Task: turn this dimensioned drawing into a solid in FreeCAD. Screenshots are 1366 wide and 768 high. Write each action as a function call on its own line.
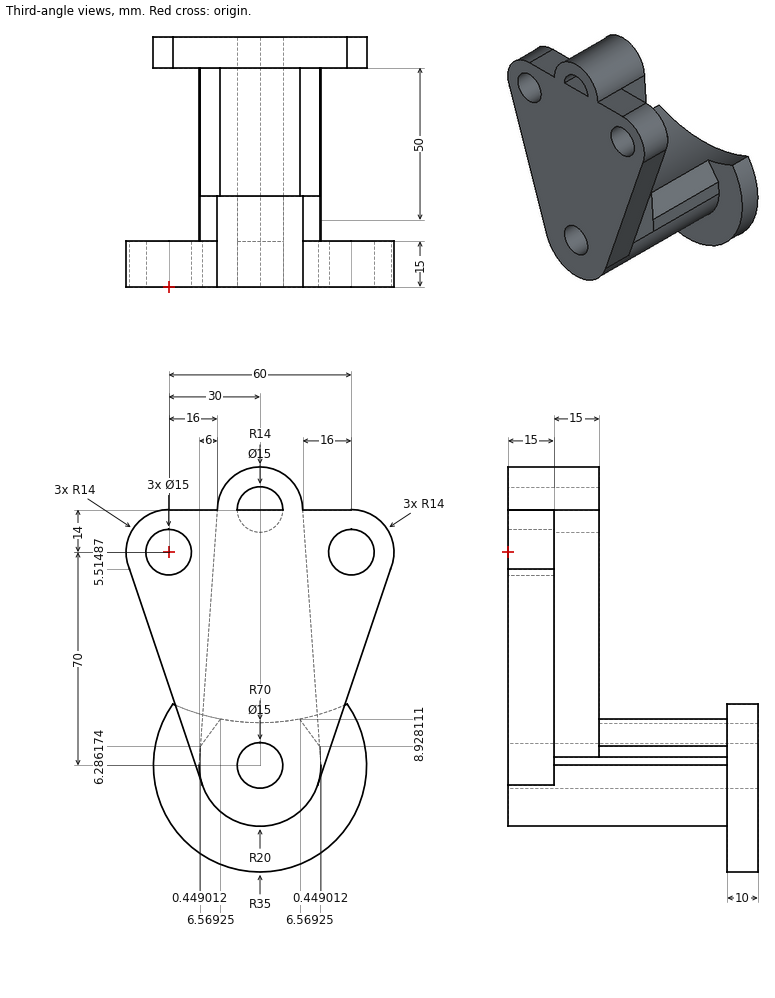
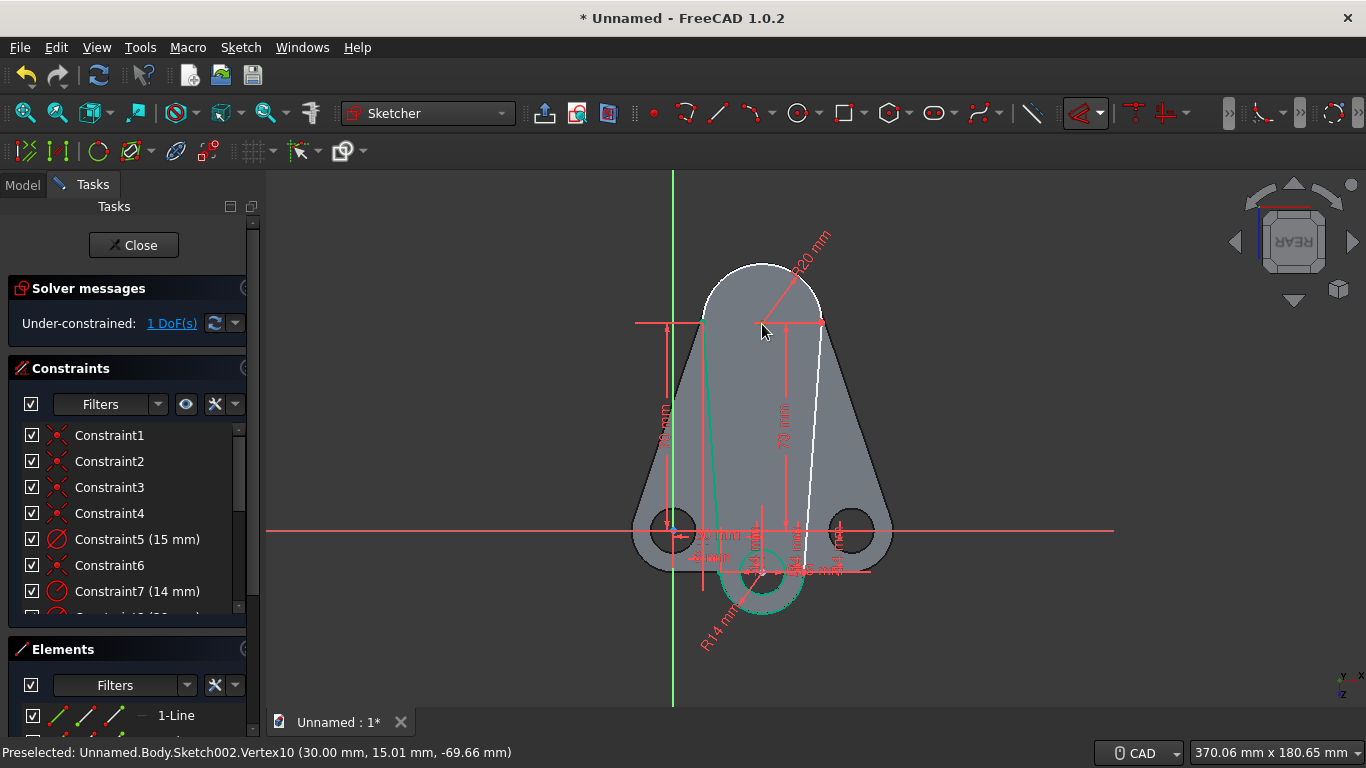
click(1102, 114)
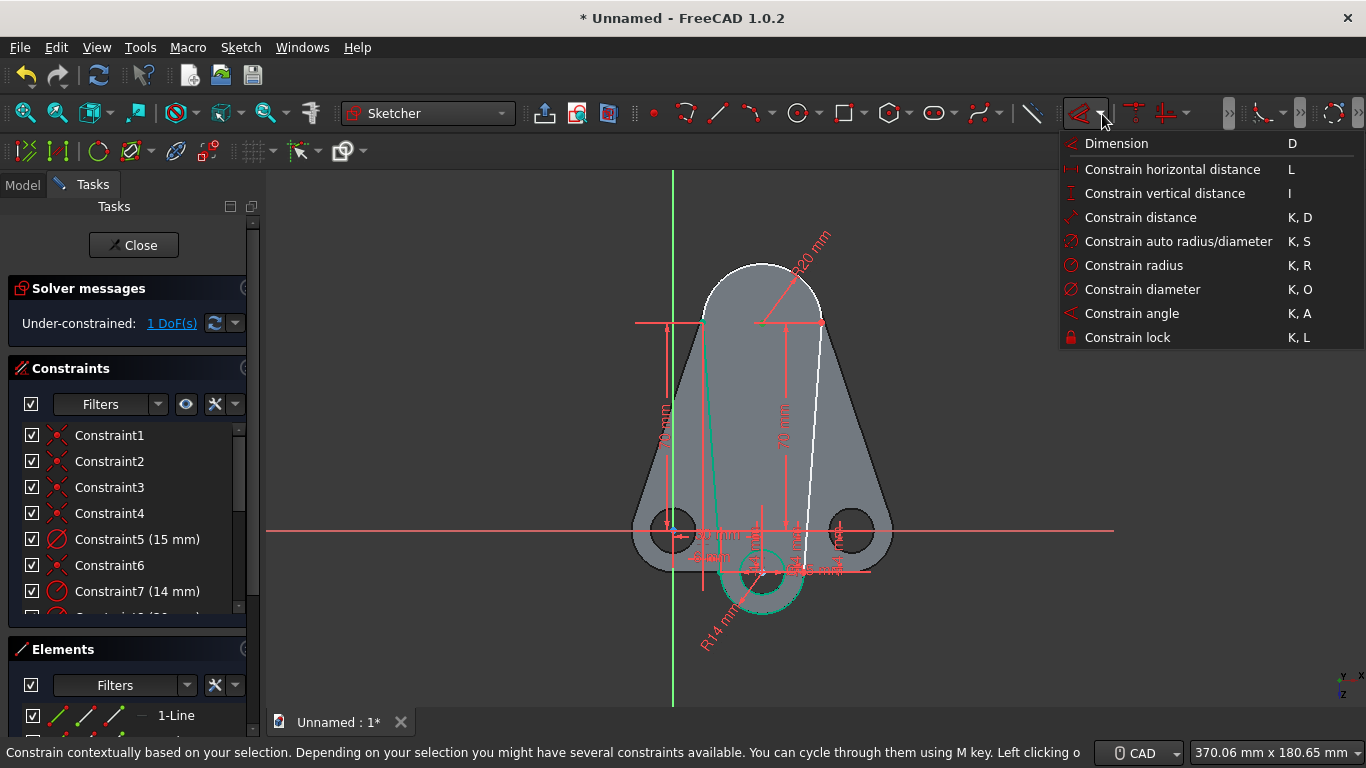
click(1212, 193)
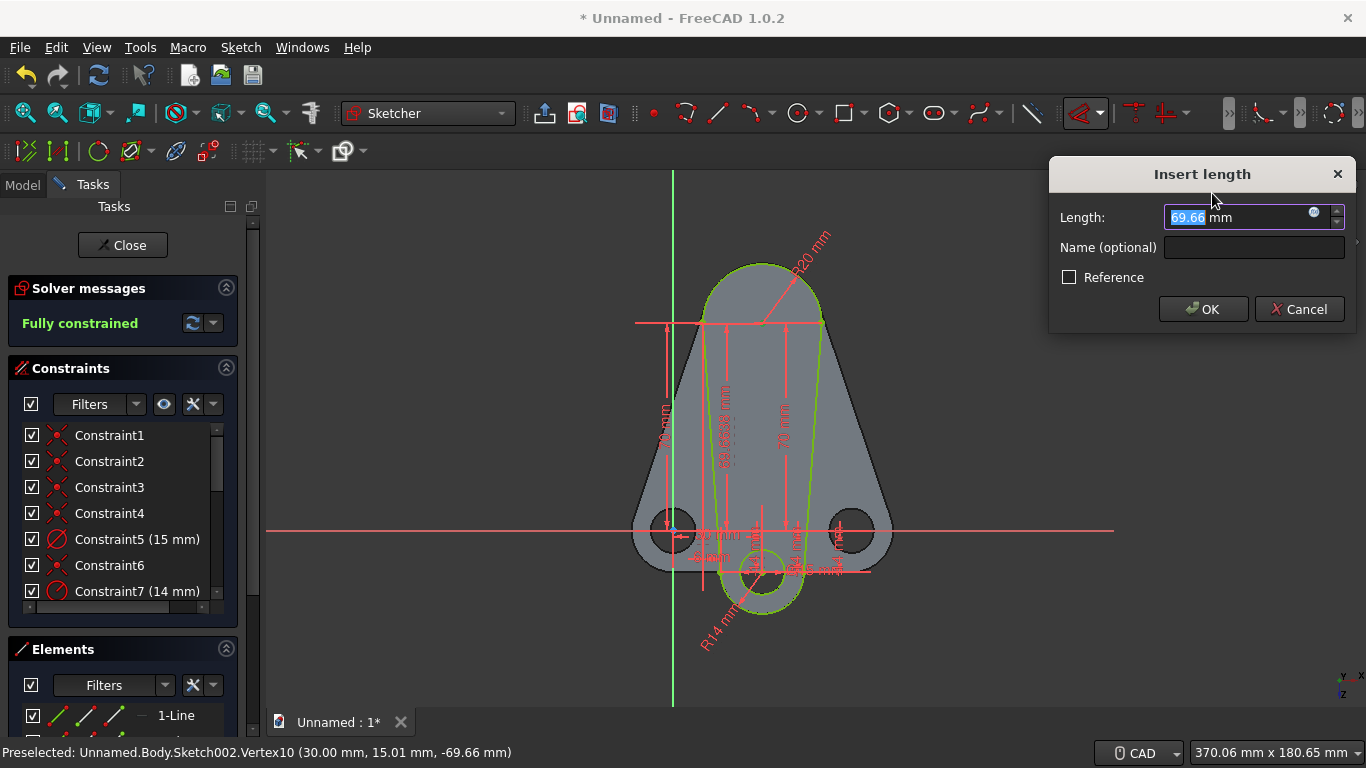
text(70)
key(Return)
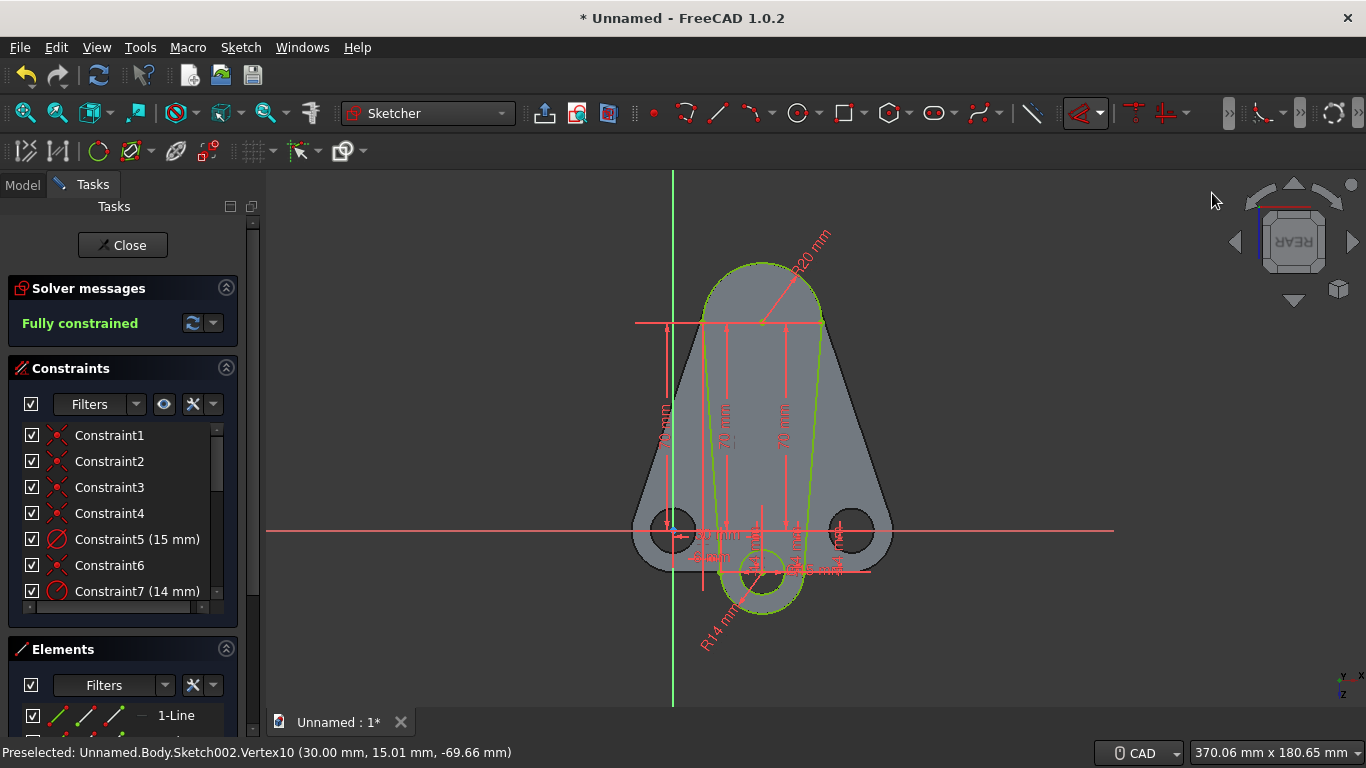
click(123, 245)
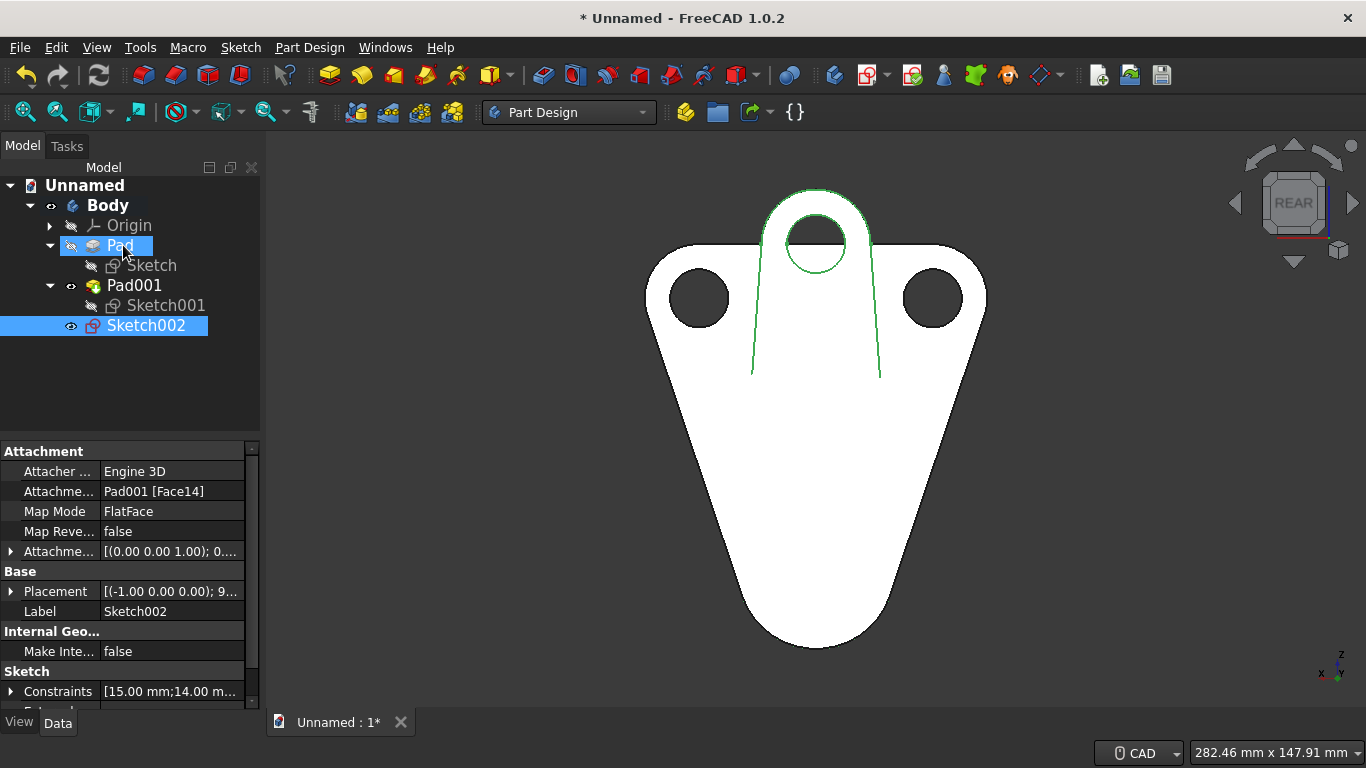
click(330, 76)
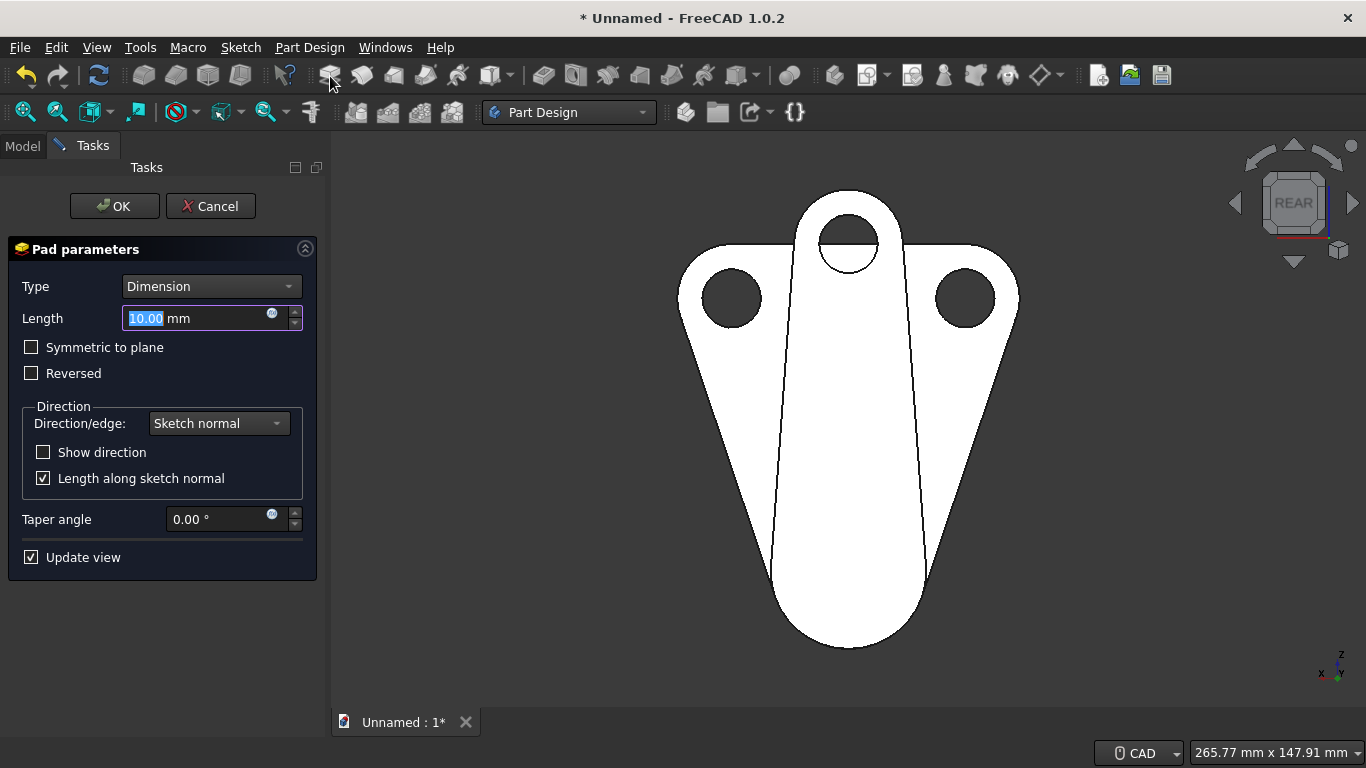
text(15)
key(Tab)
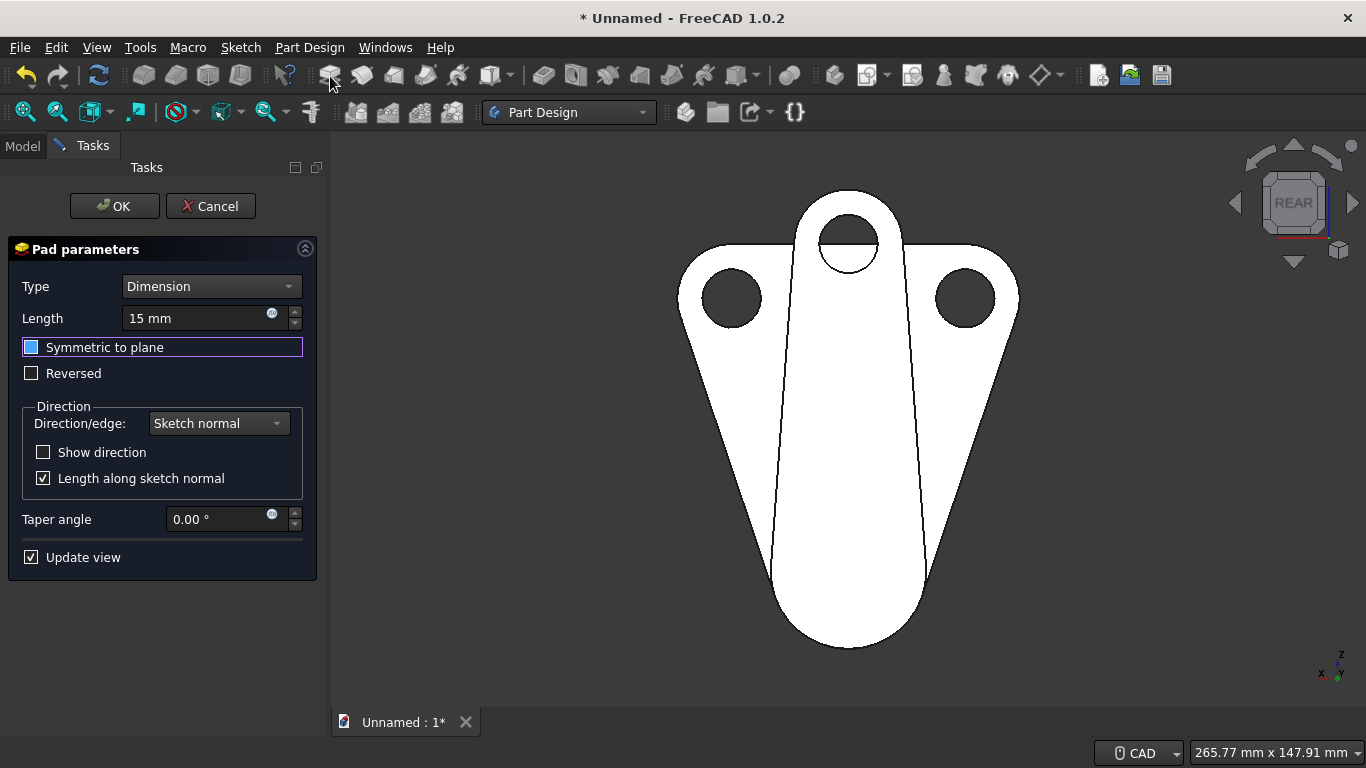
click(115, 206)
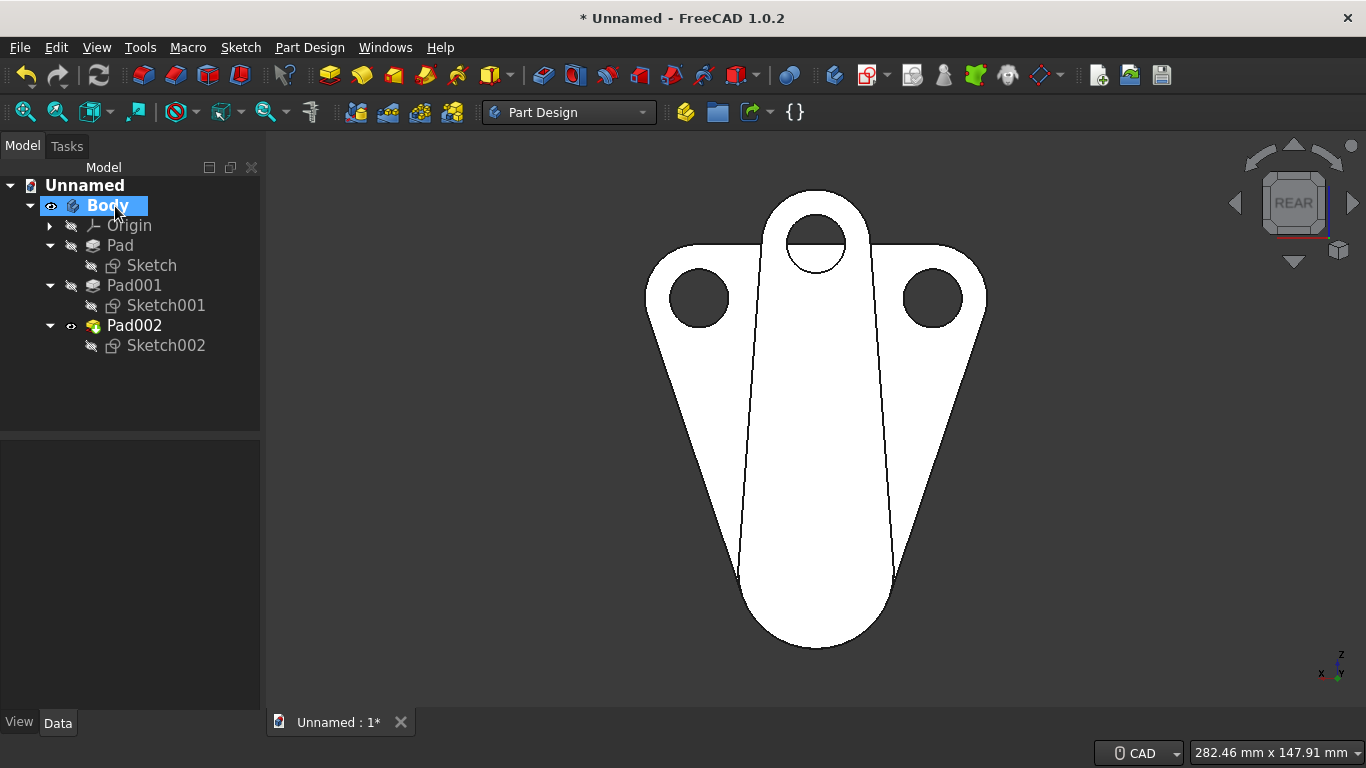
click(50, 226)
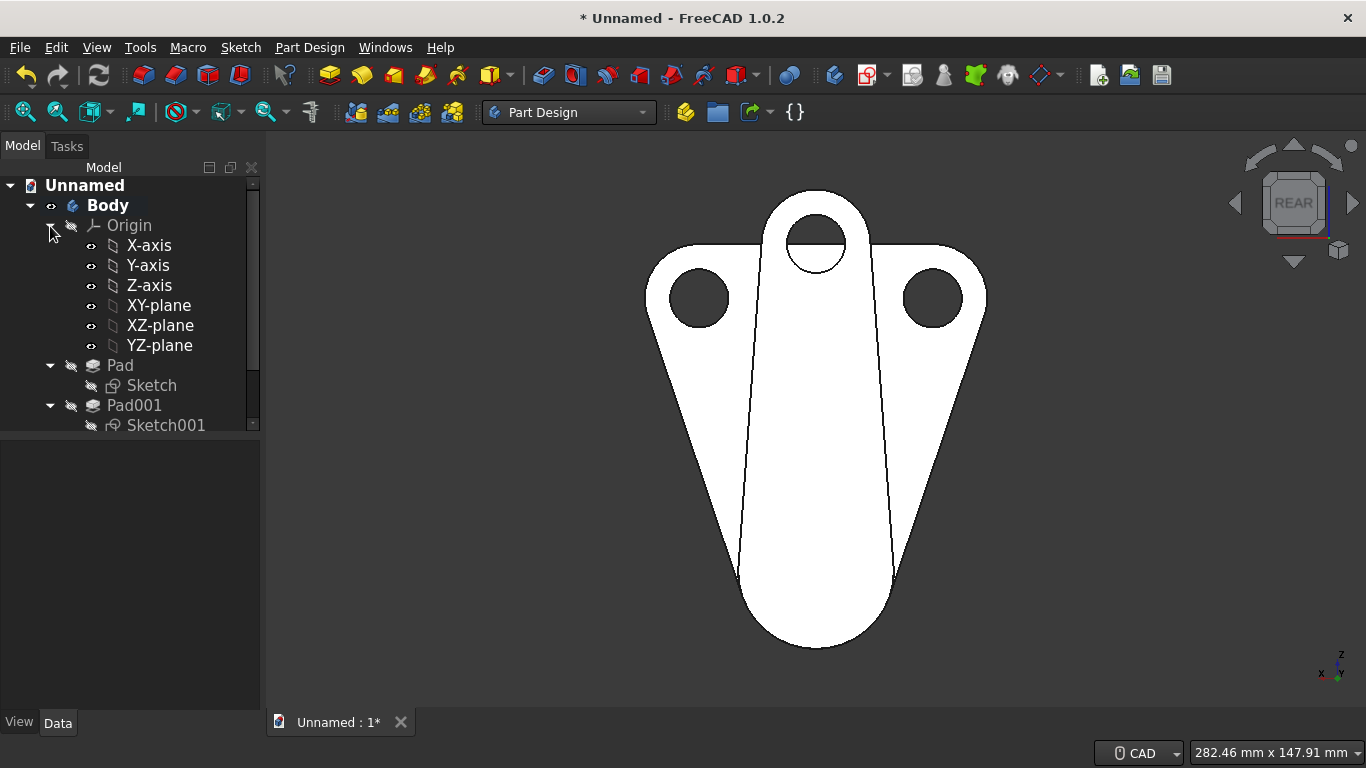
click(136, 326)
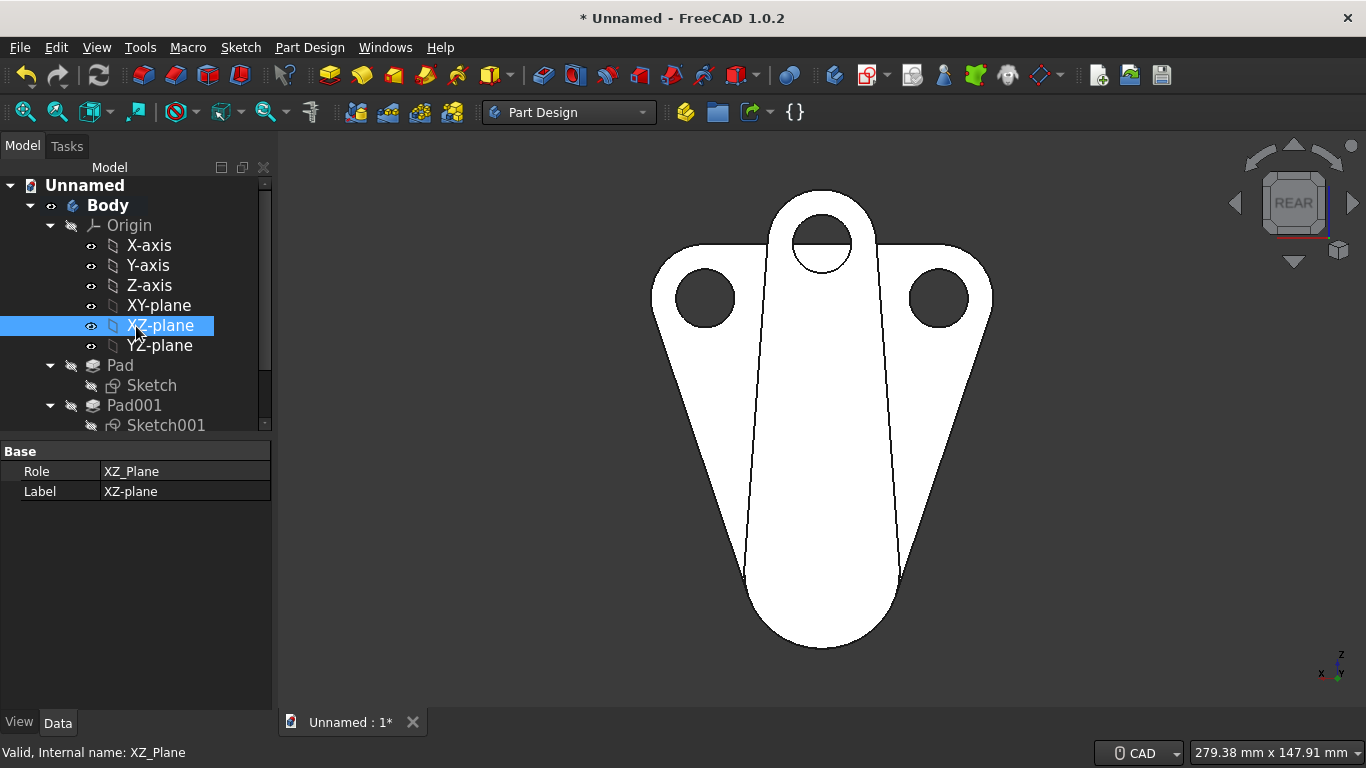
click(1040, 76)